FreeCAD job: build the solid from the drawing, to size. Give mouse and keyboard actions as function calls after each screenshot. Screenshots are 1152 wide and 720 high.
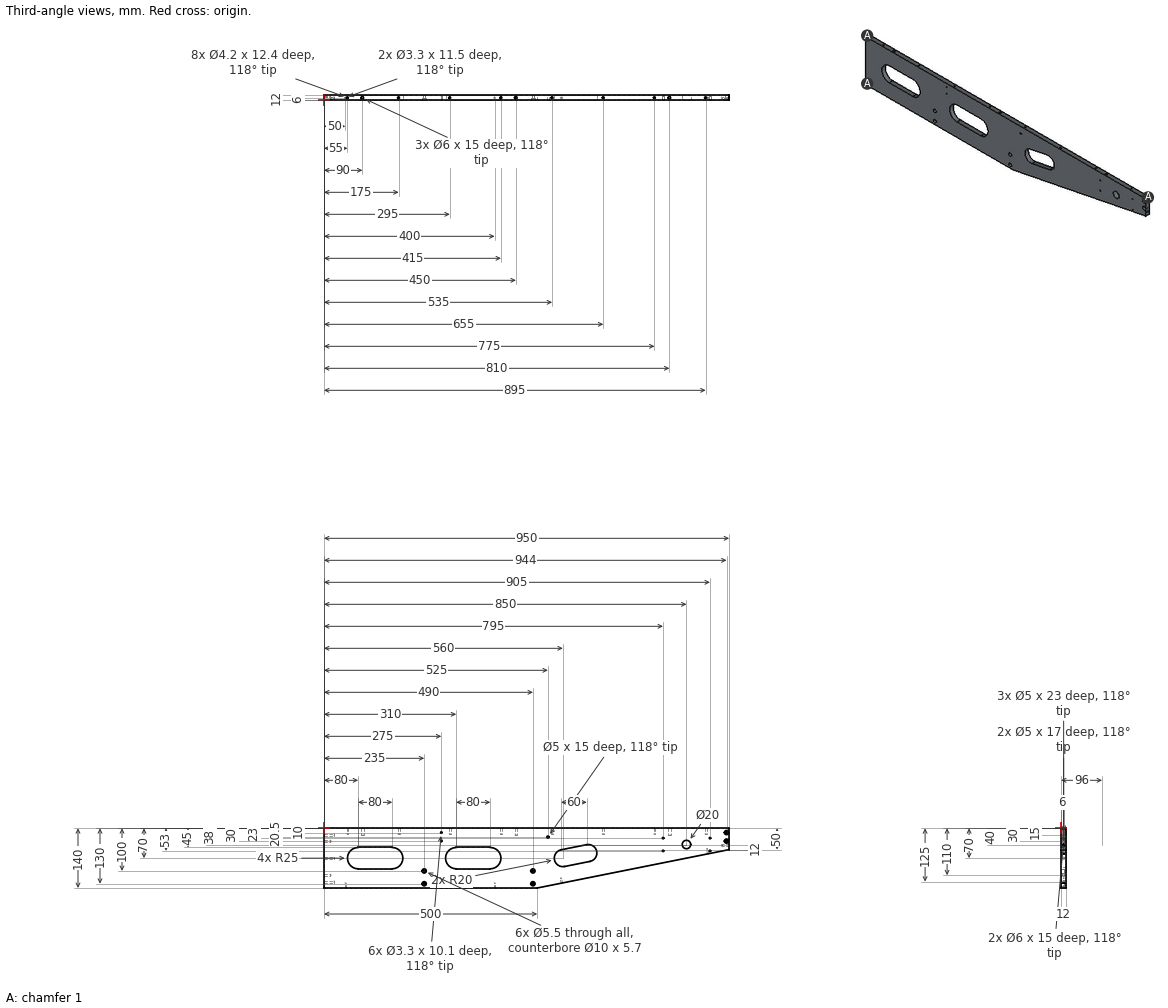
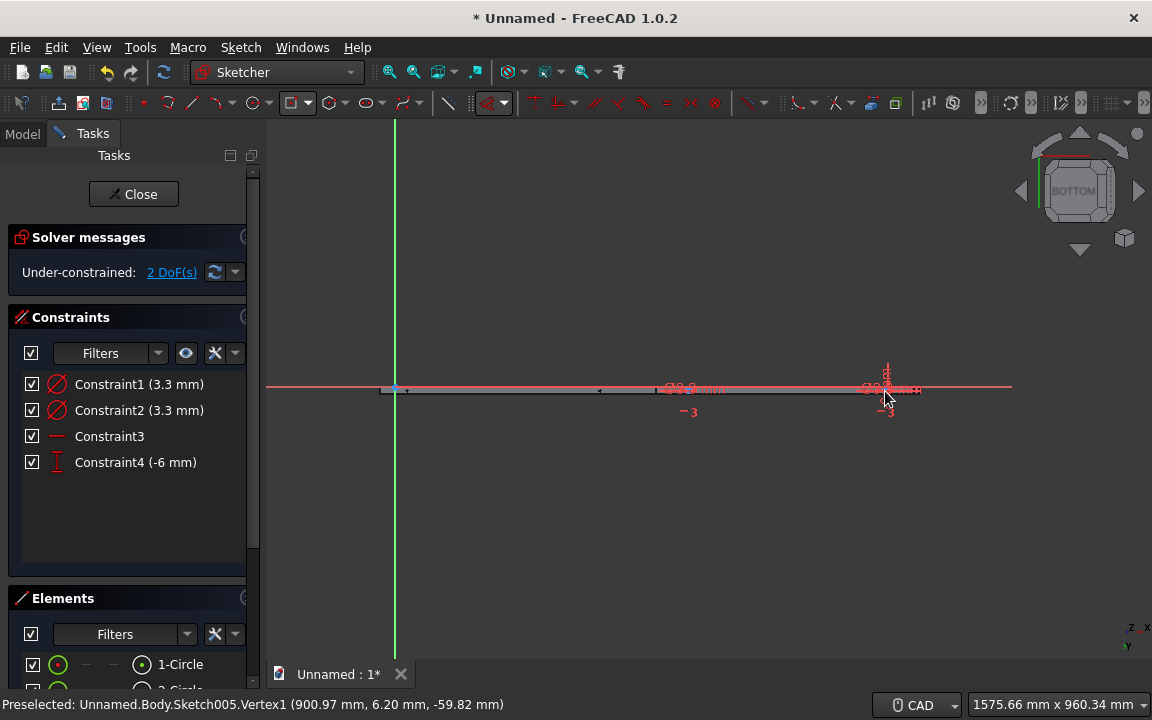
click(885, 391)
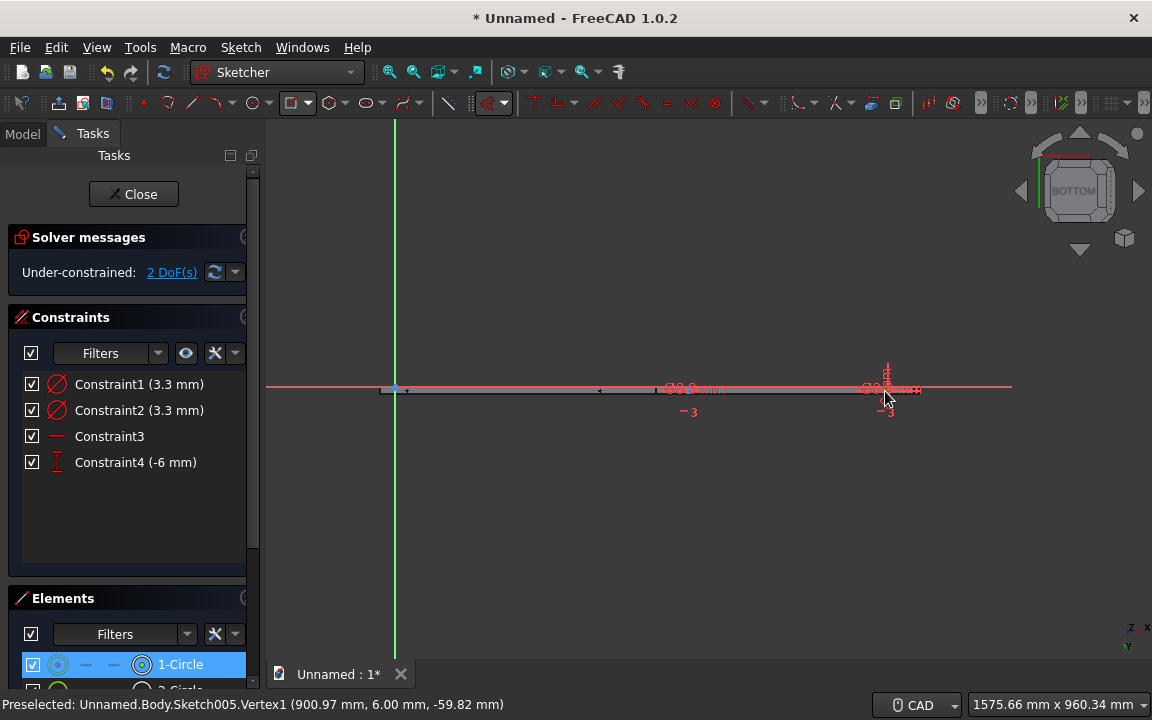
click(689, 391)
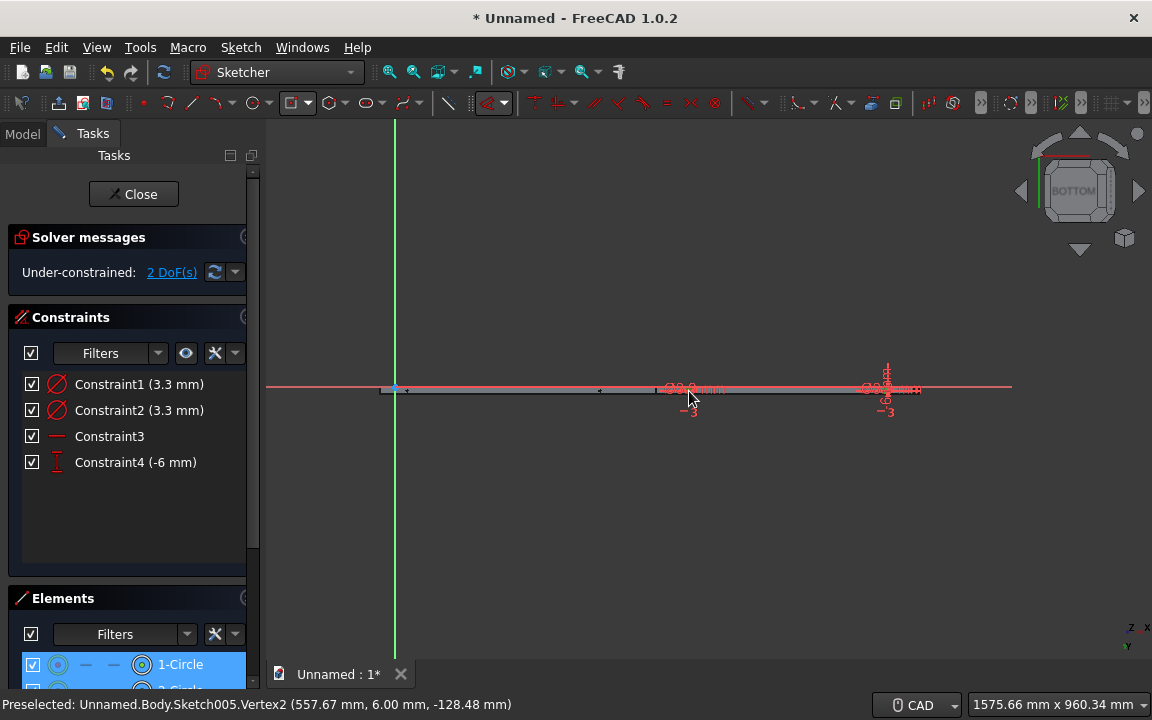
key(l)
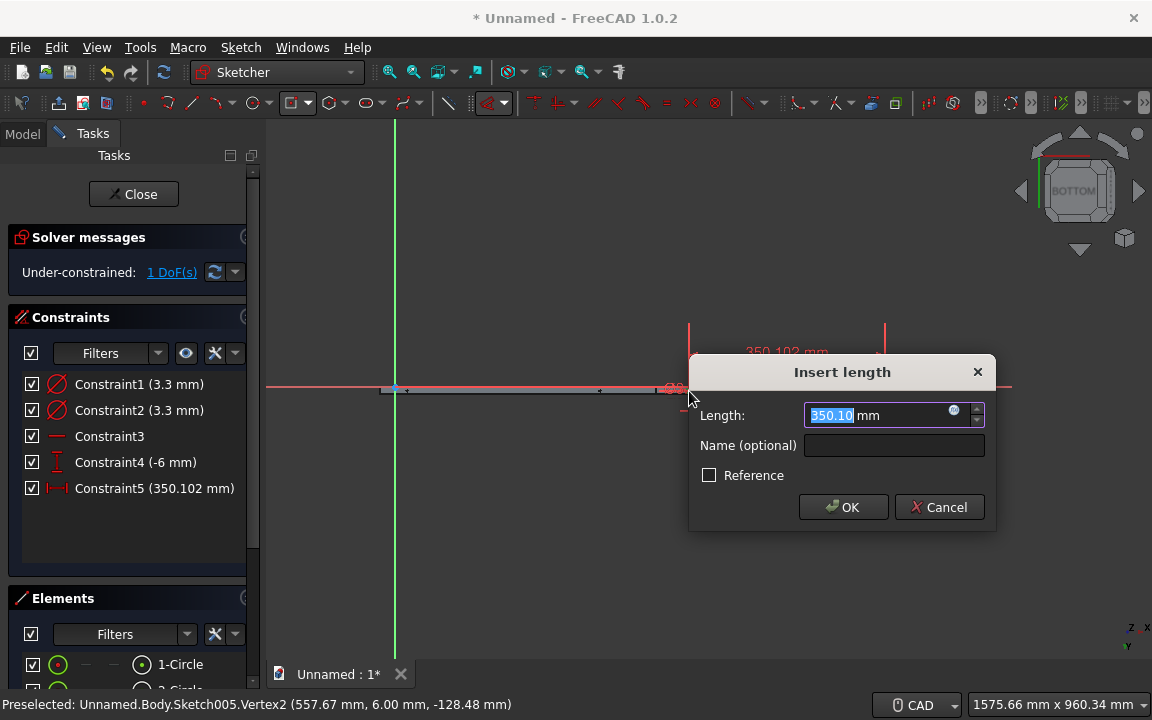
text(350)
key(Return)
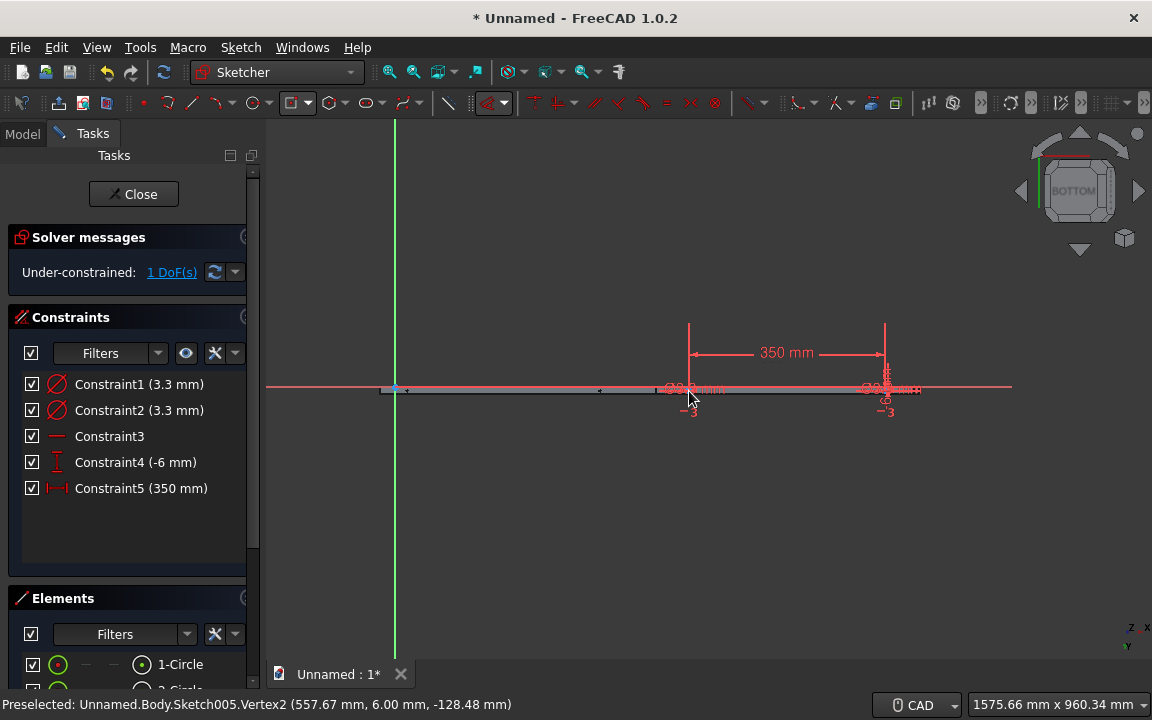
click(885, 391)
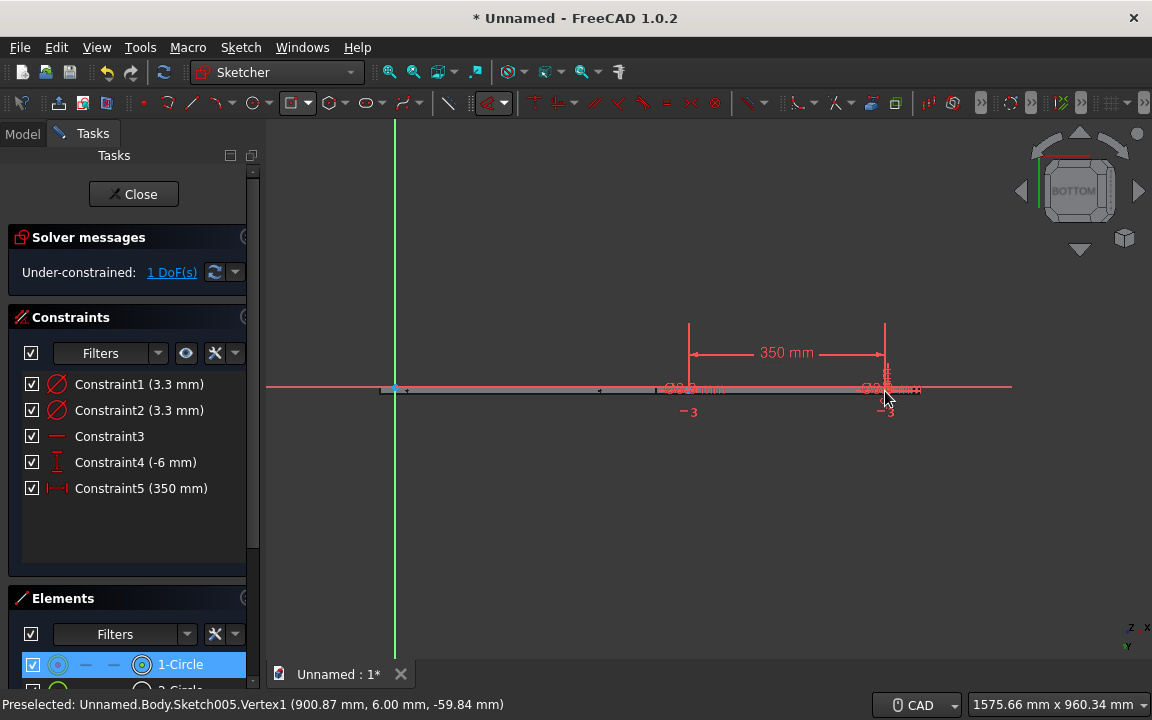
click(506, 104)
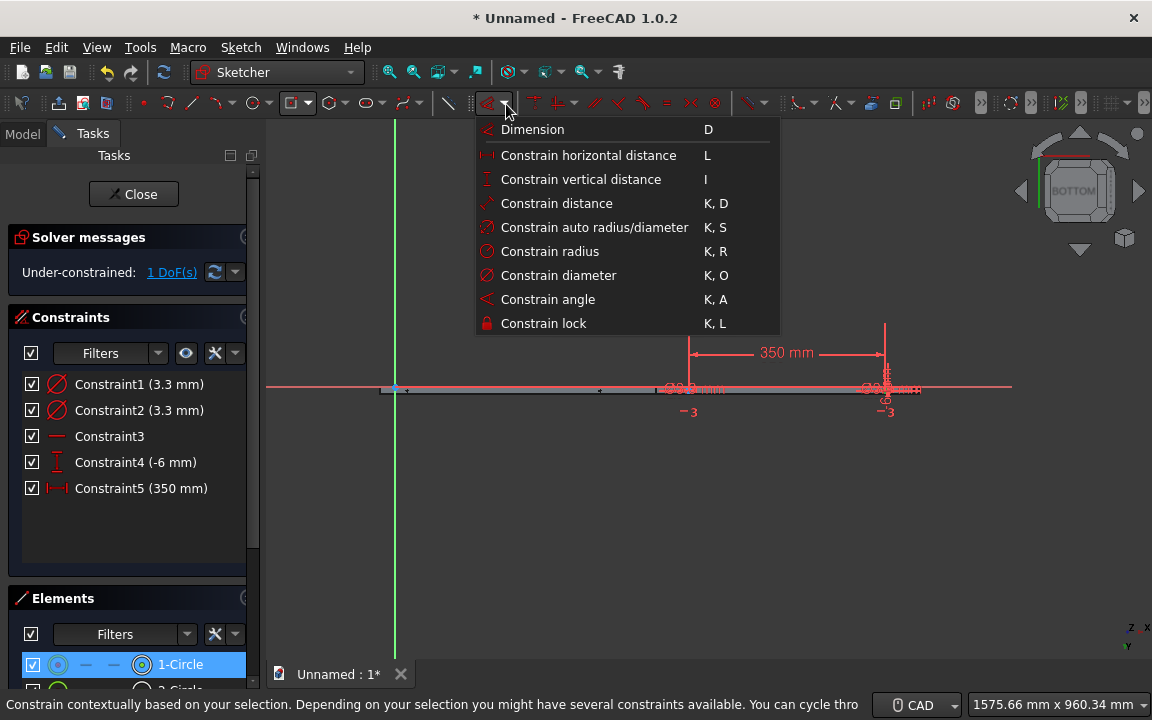
click(628, 155)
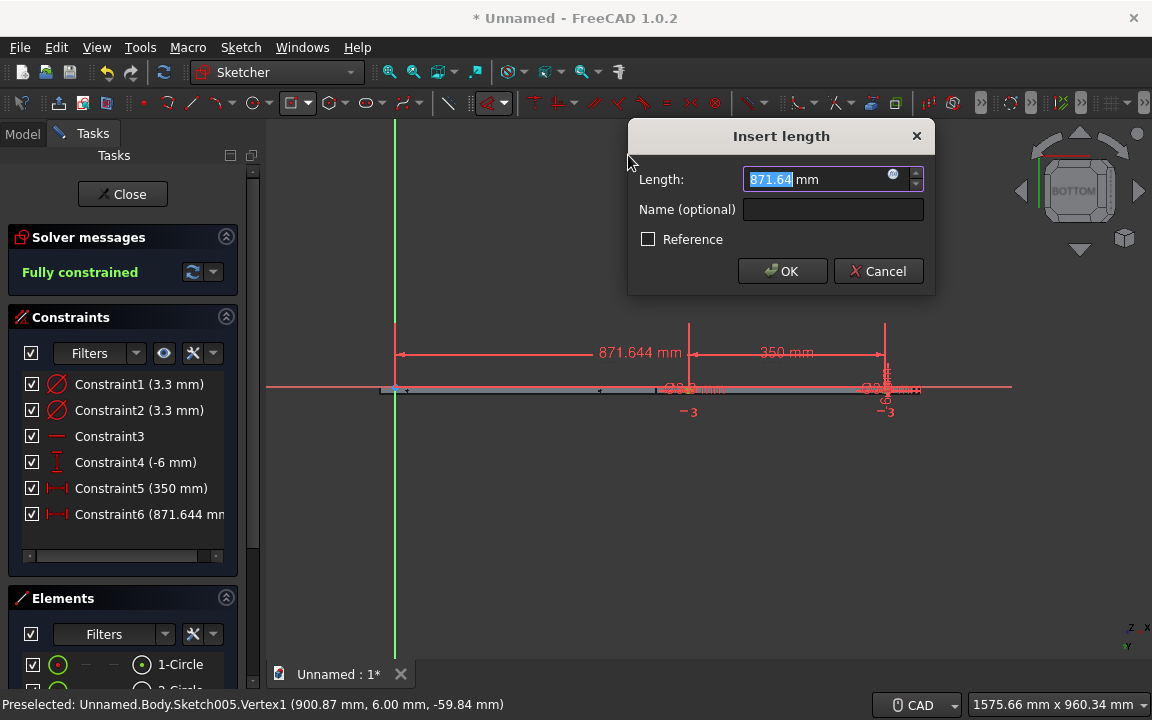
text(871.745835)
key(Return)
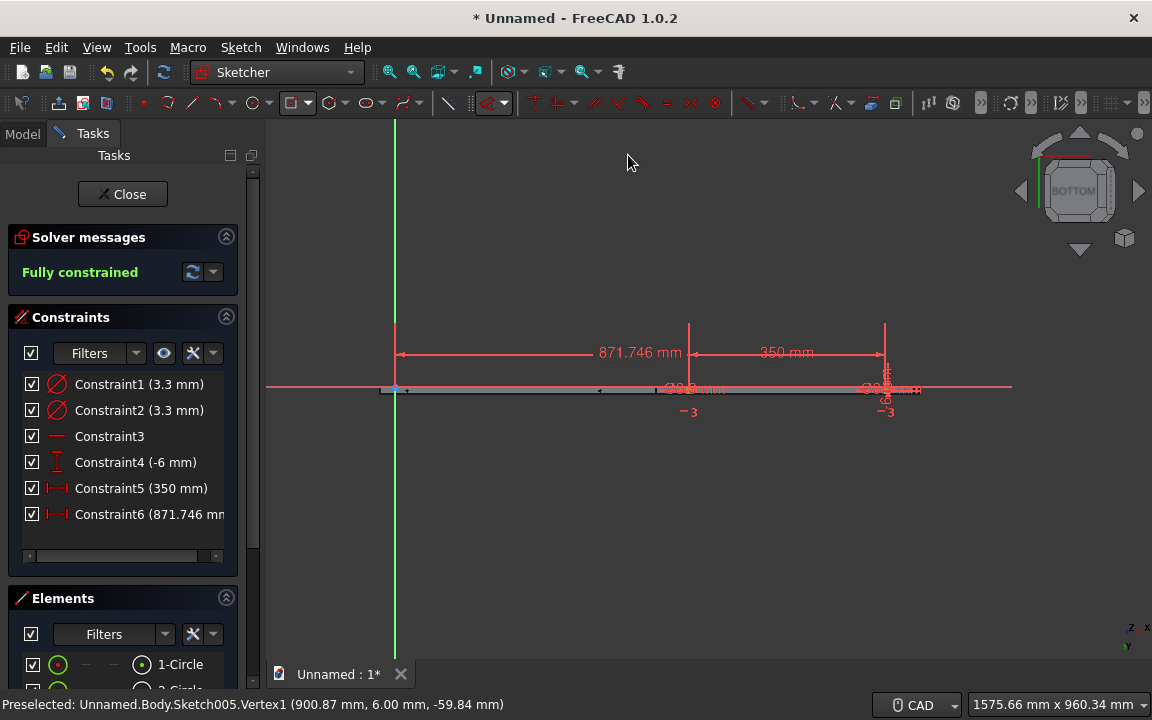
click(123, 194)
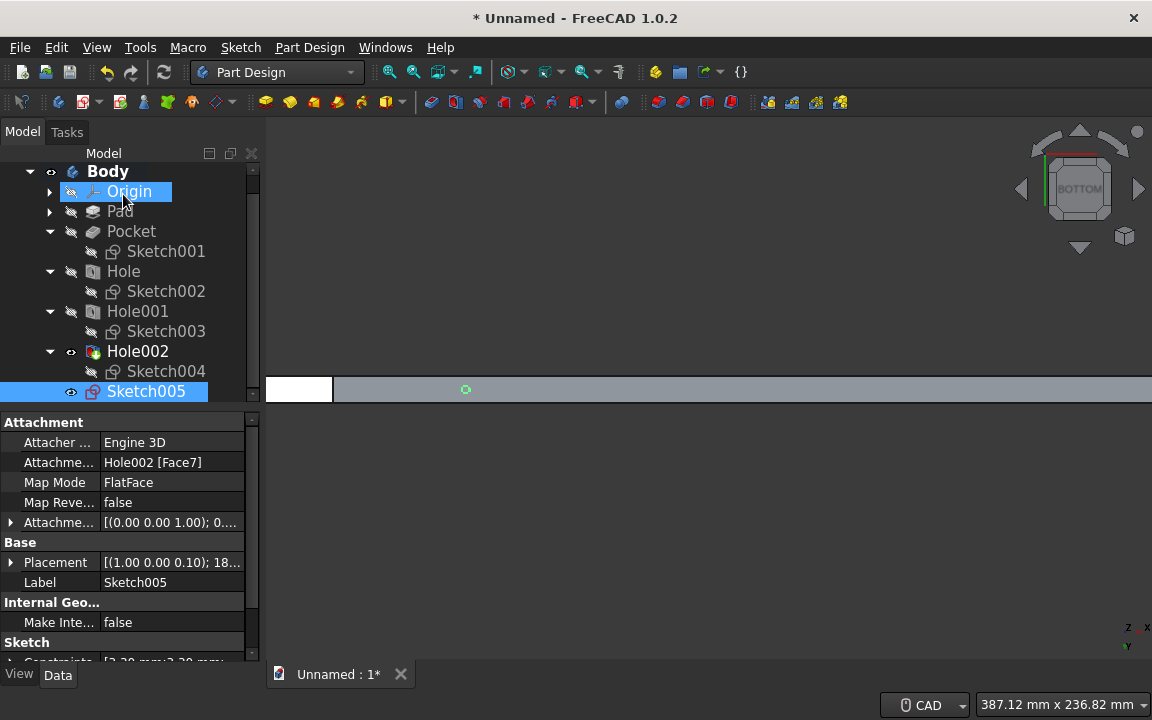
click(456, 102)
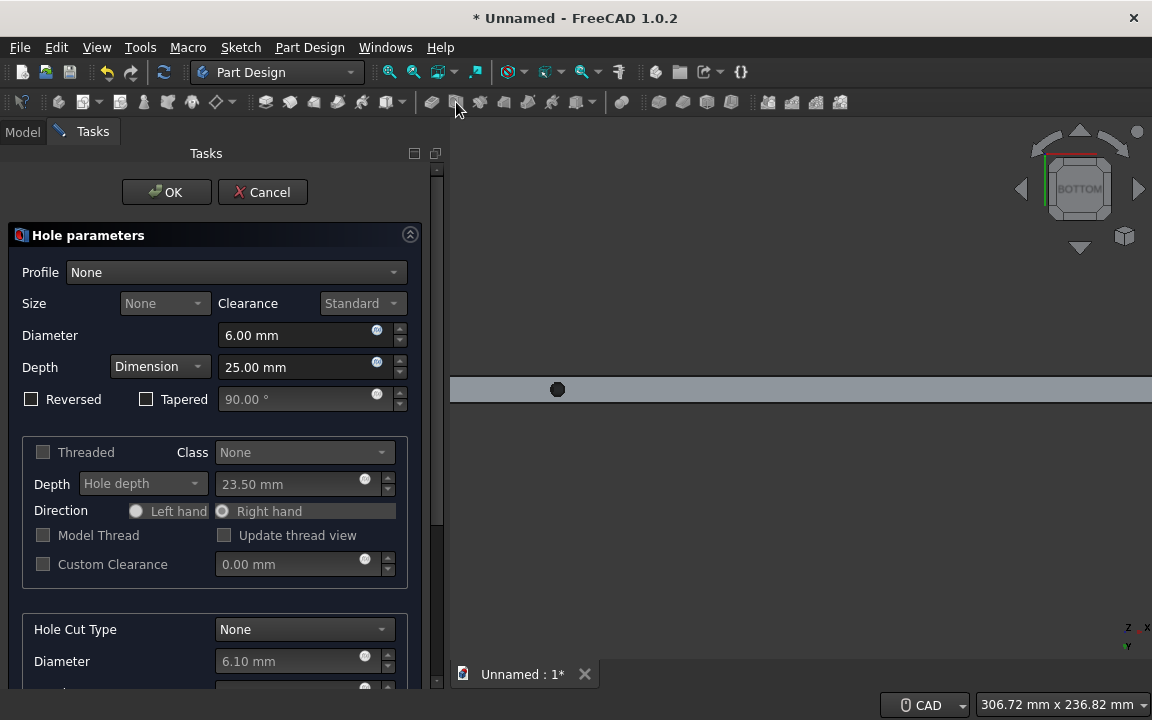
triple_click(305, 335)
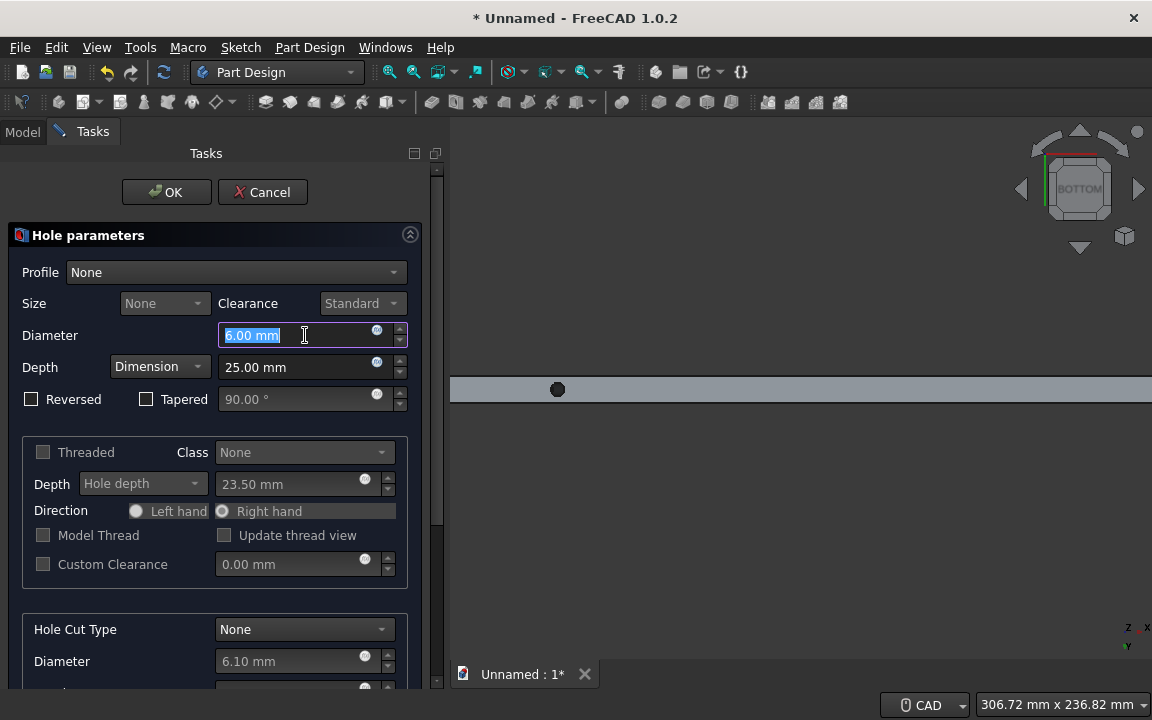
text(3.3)
key(Tab)